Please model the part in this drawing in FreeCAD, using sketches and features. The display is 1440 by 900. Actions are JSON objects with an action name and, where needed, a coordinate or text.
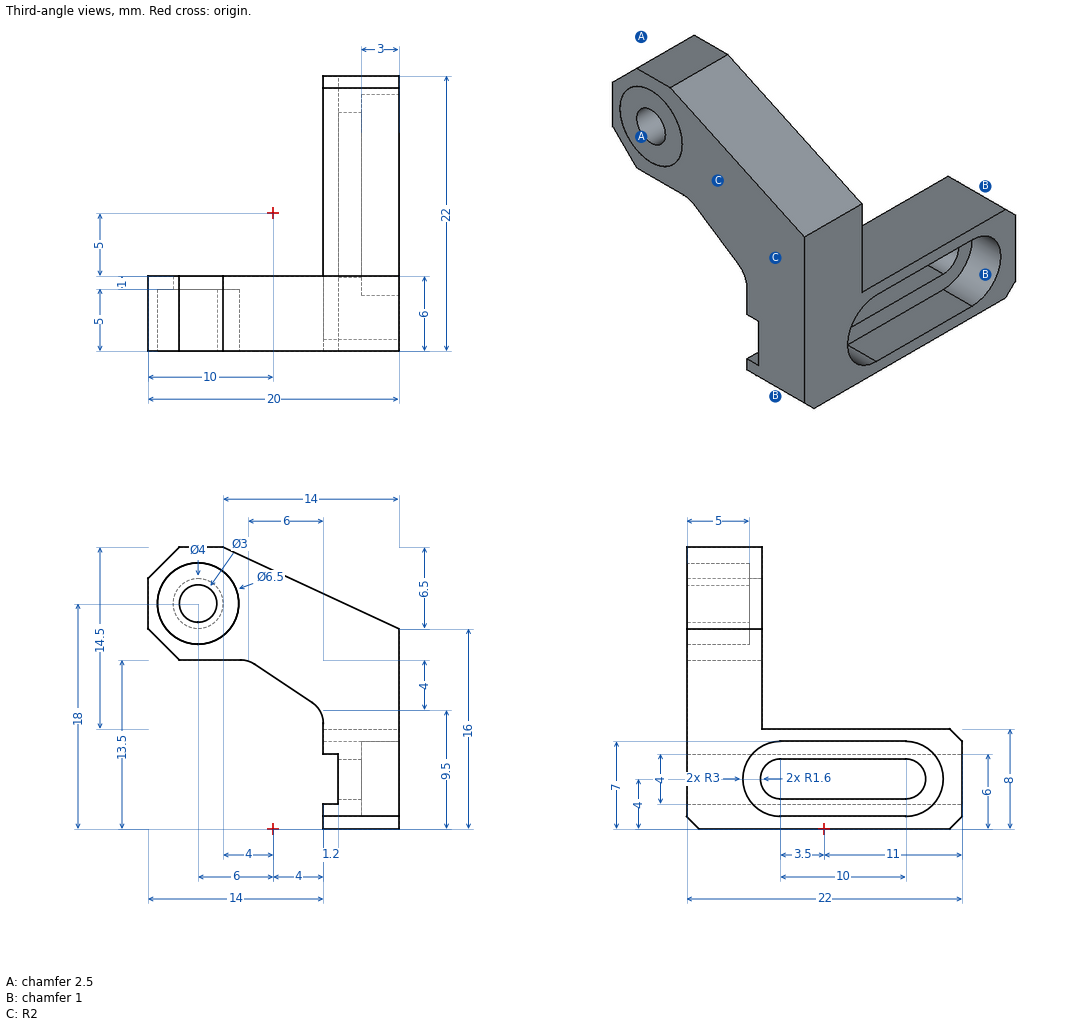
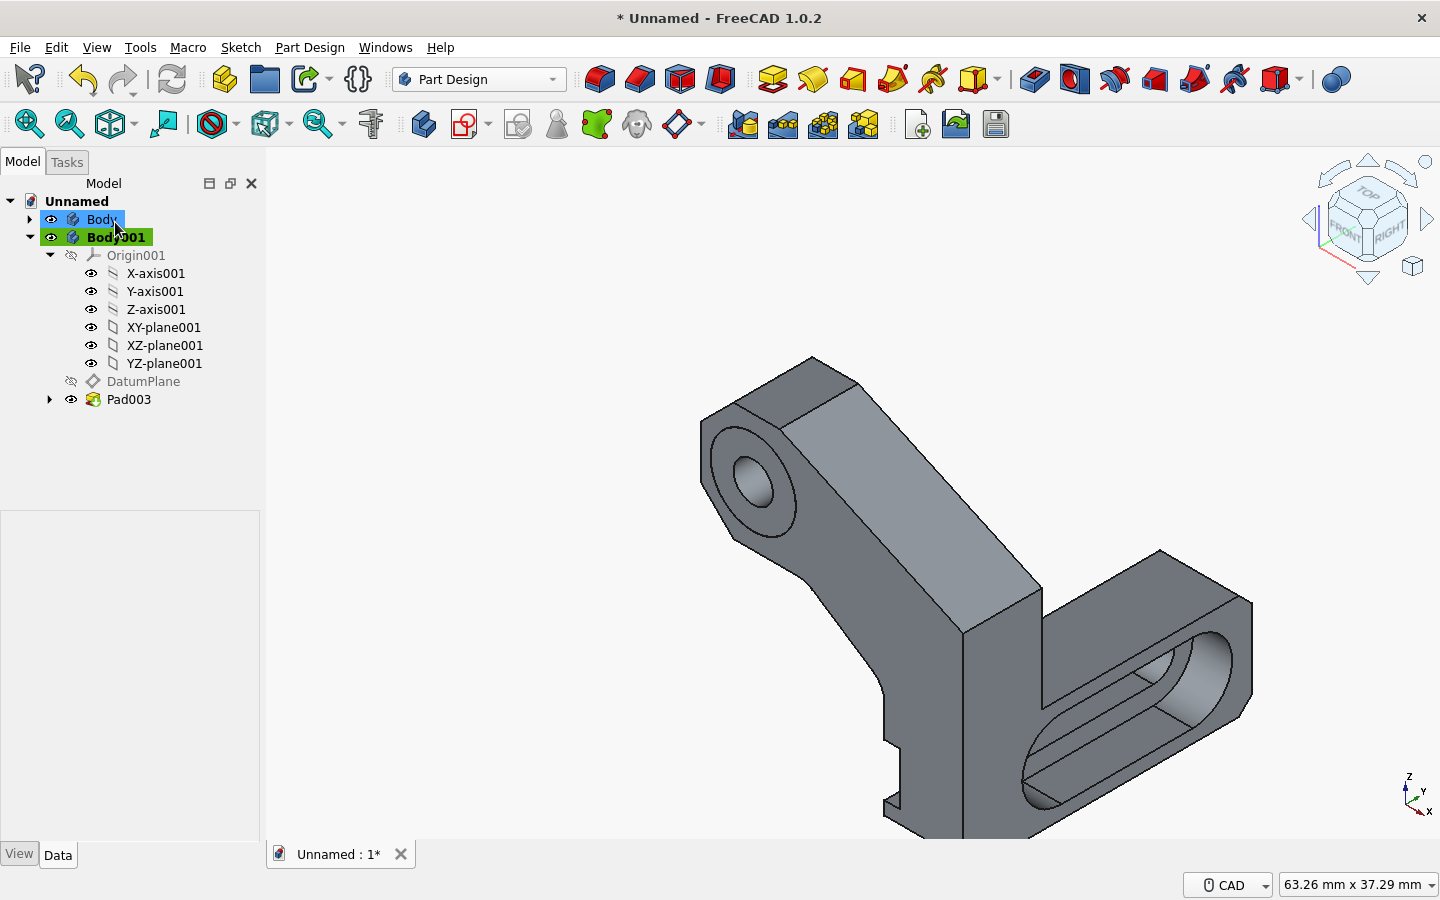
{"action": "left_click", "coordinate": [30, 124]}